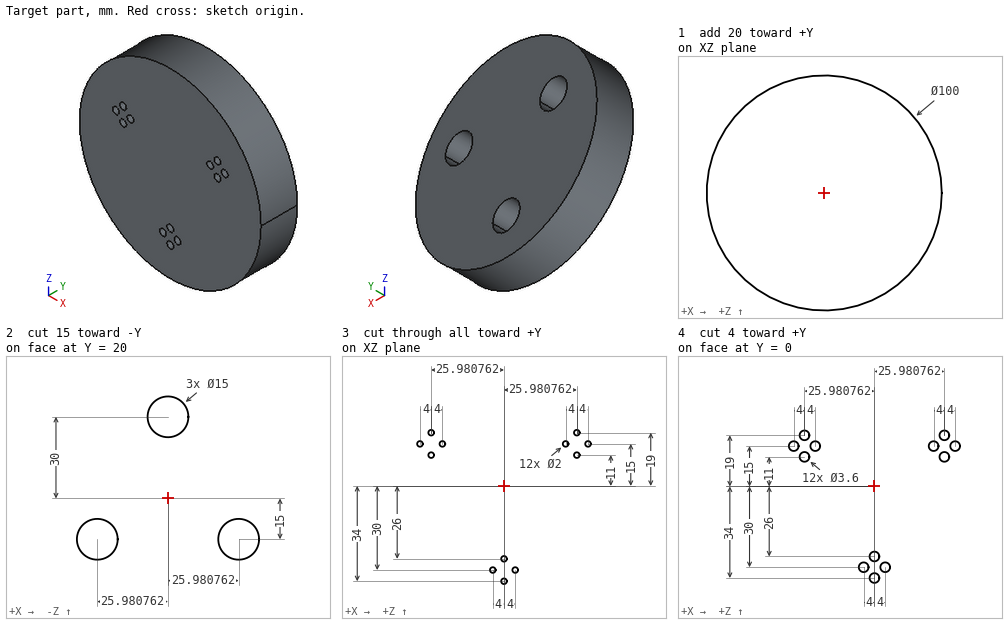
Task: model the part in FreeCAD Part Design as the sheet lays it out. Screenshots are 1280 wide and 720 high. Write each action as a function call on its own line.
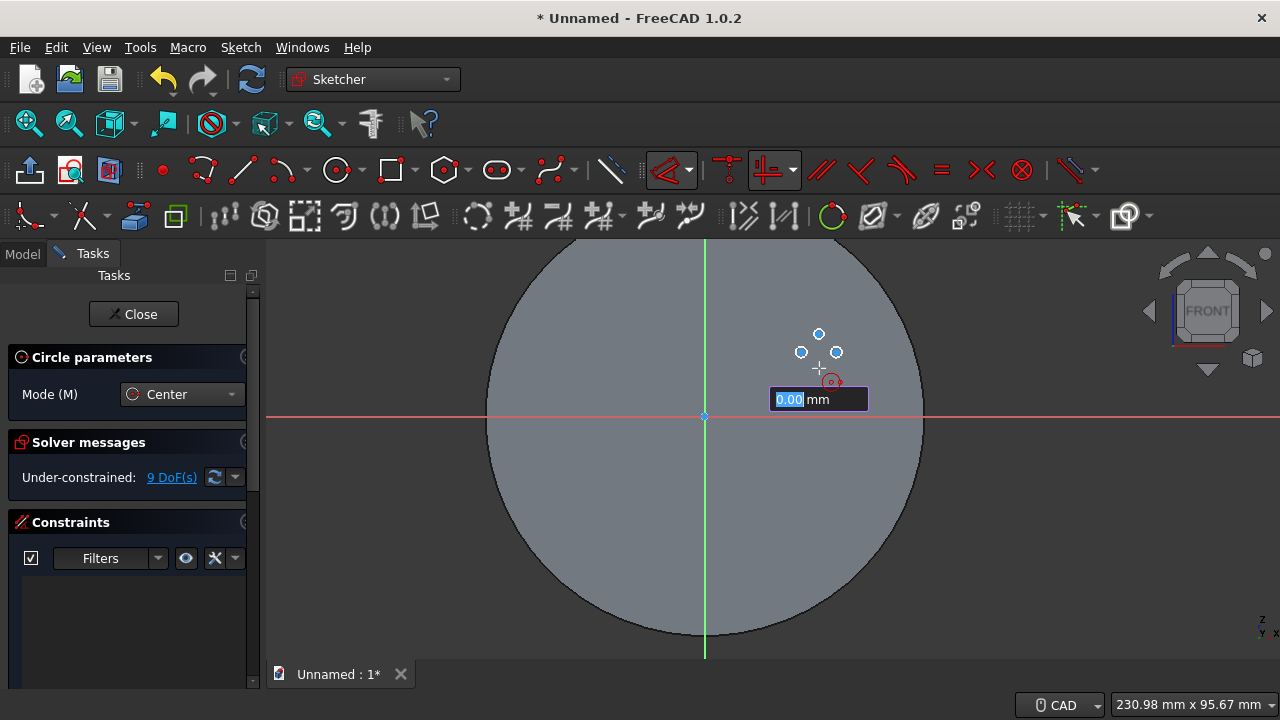
scroll(822, 365, up, 7)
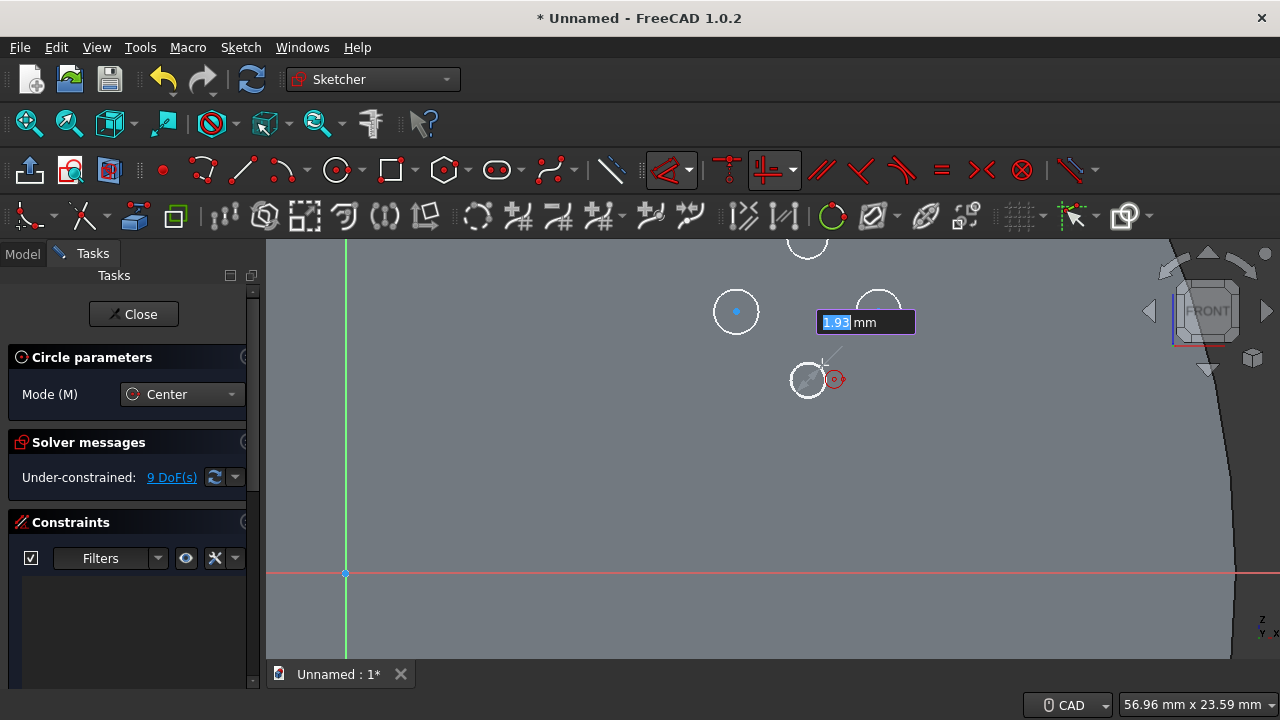
click(821, 365)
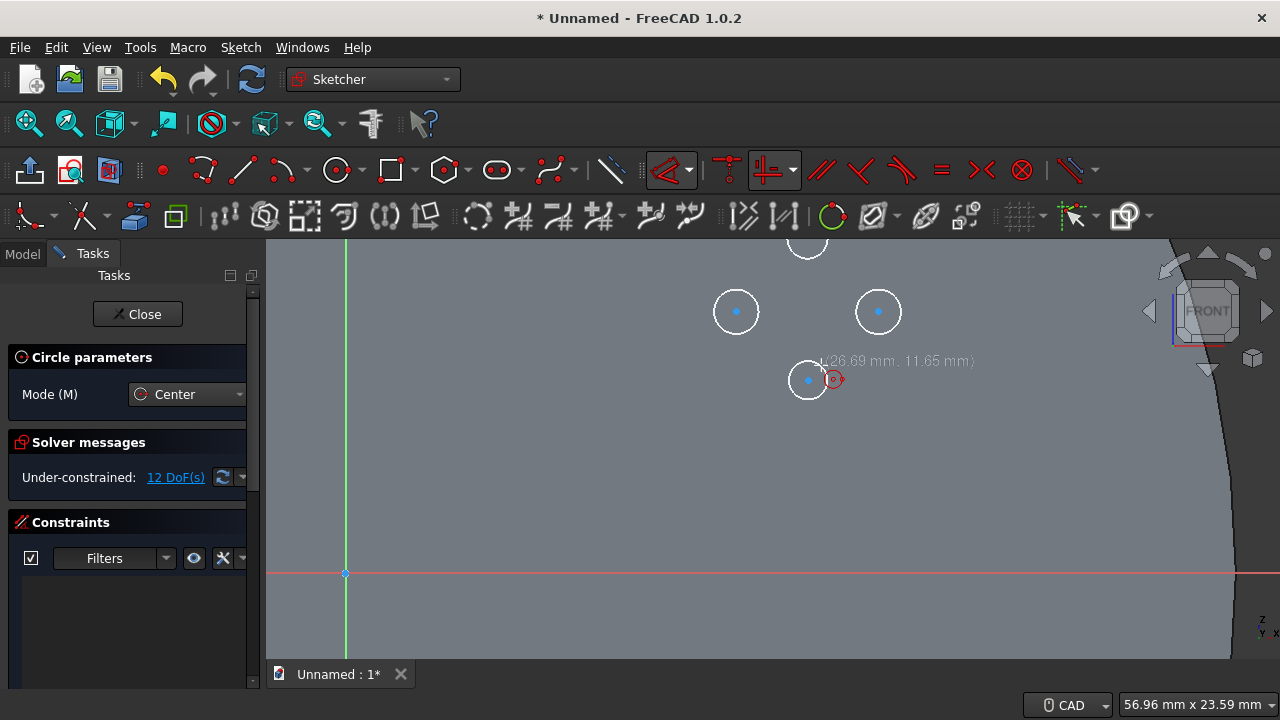
scroll(822, 365, down, 7)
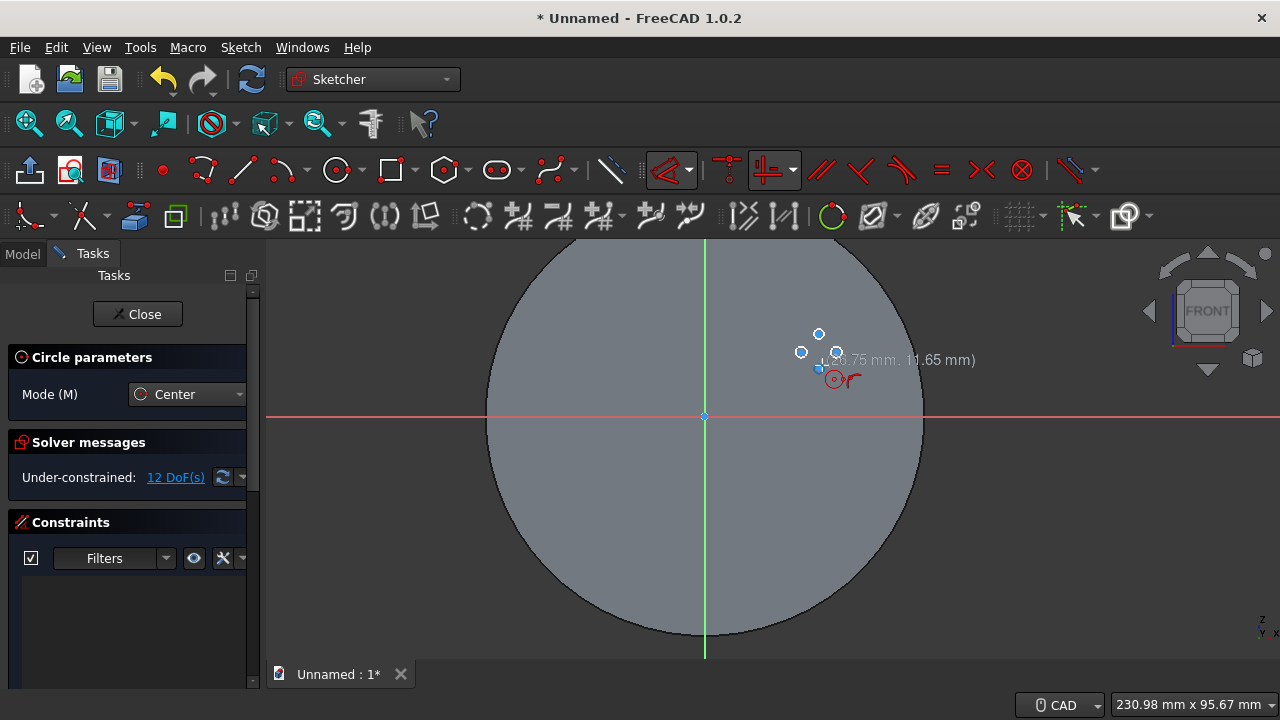
scroll(591, 333, up, 9)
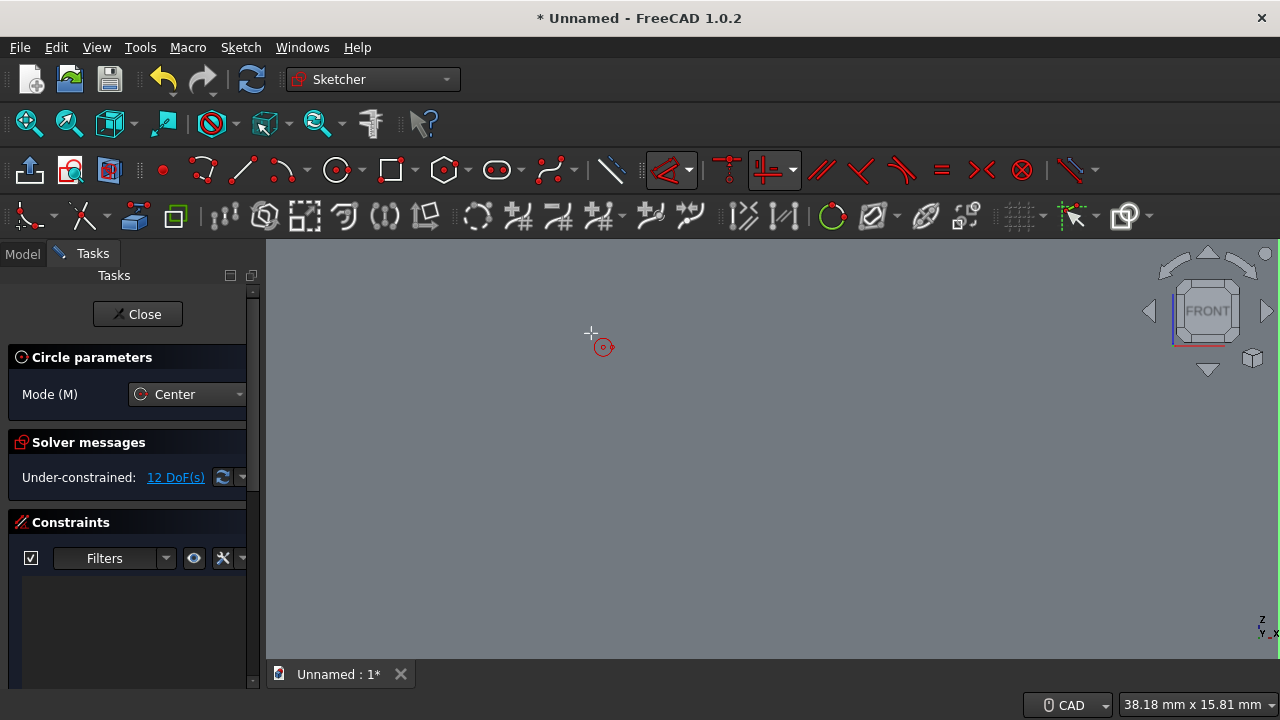
scroll(591, 333, down, 9)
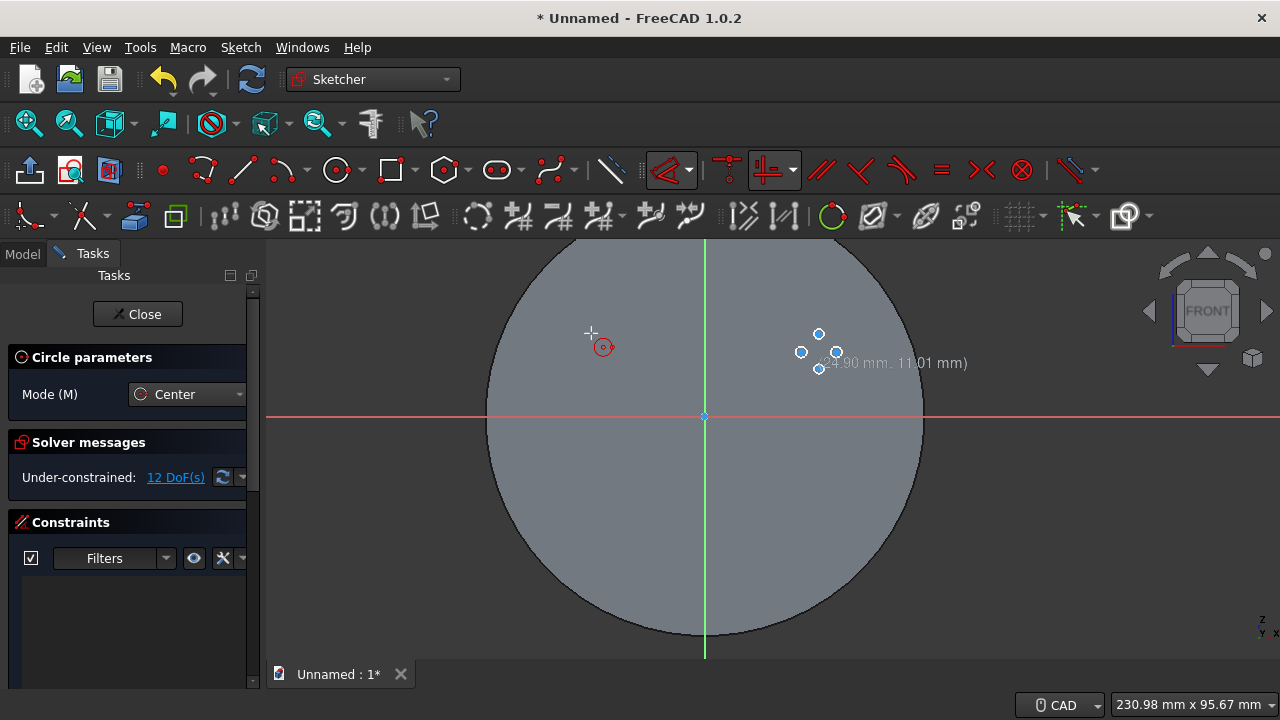
click(591, 333)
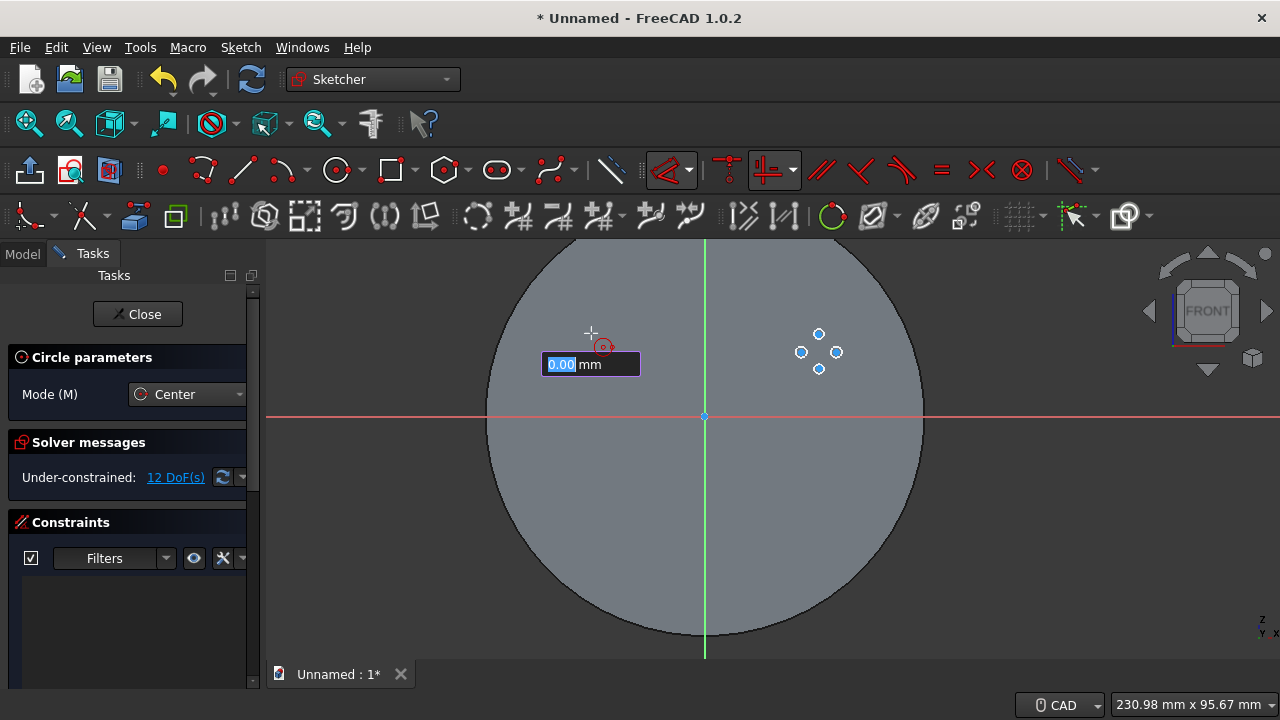
scroll(594, 330, up, 7)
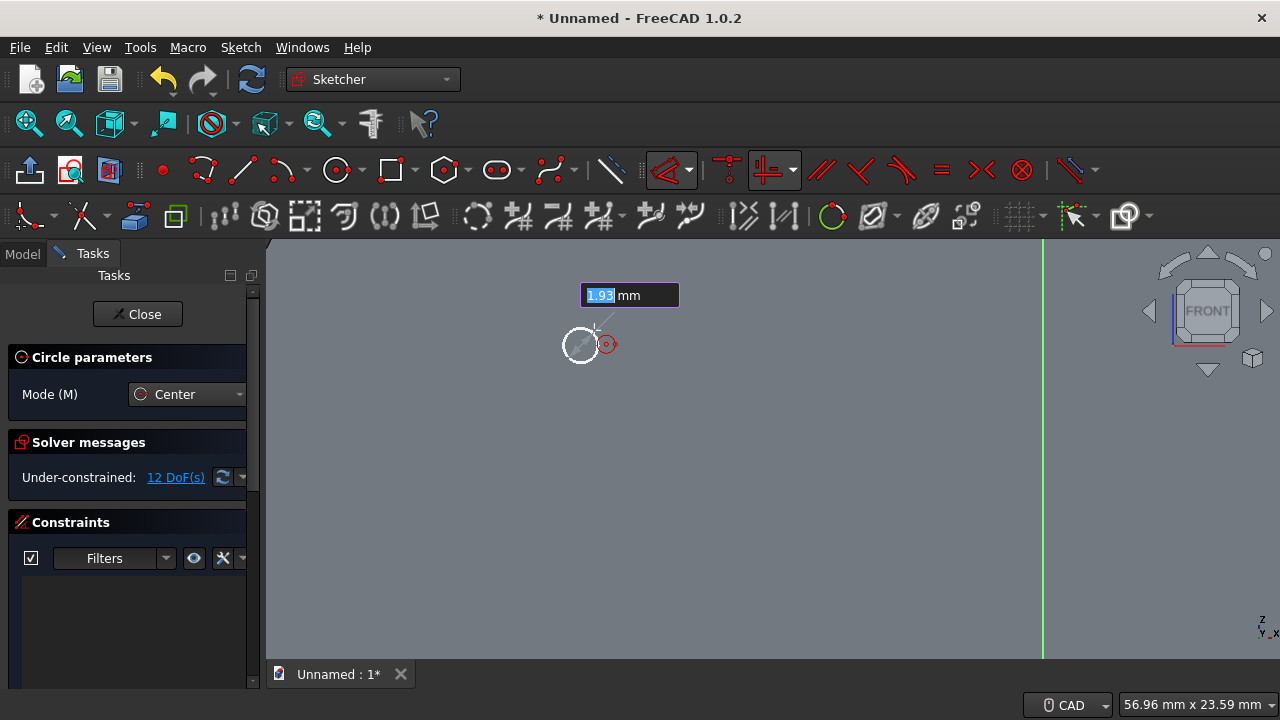
click(593, 330)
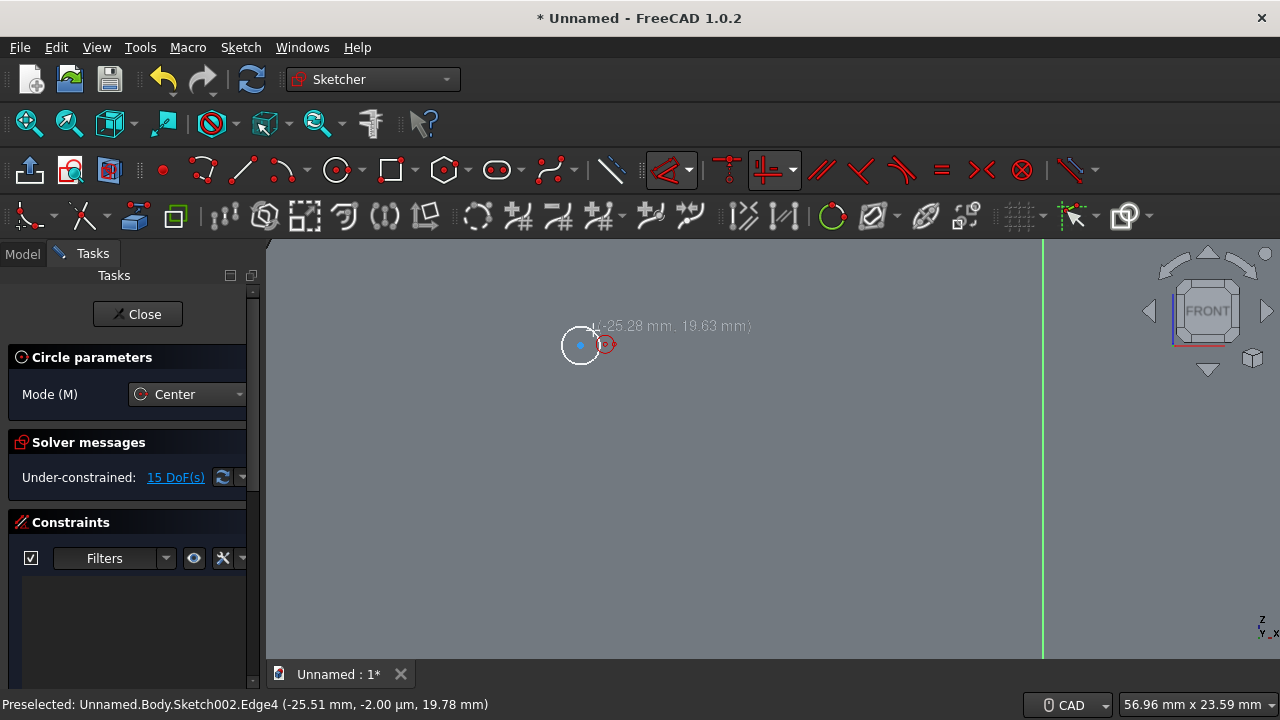
scroll(509, 413, up, 2)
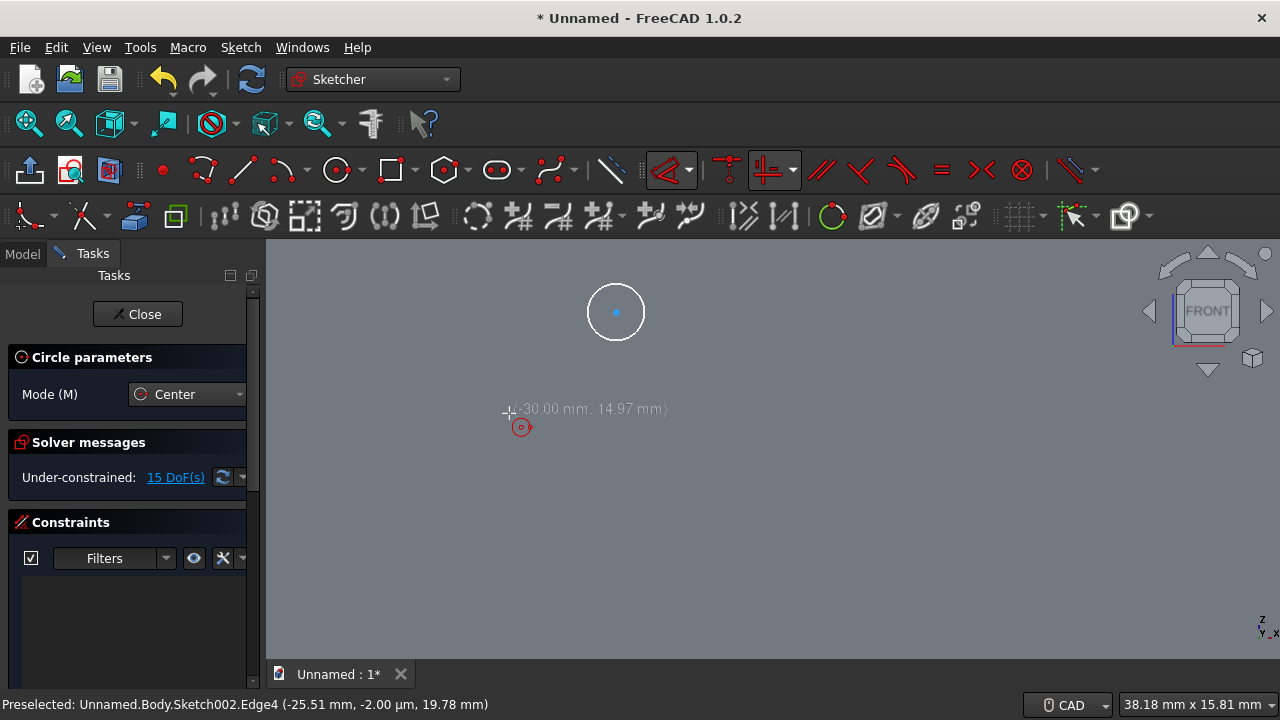
scroll(585, 338, down, 9)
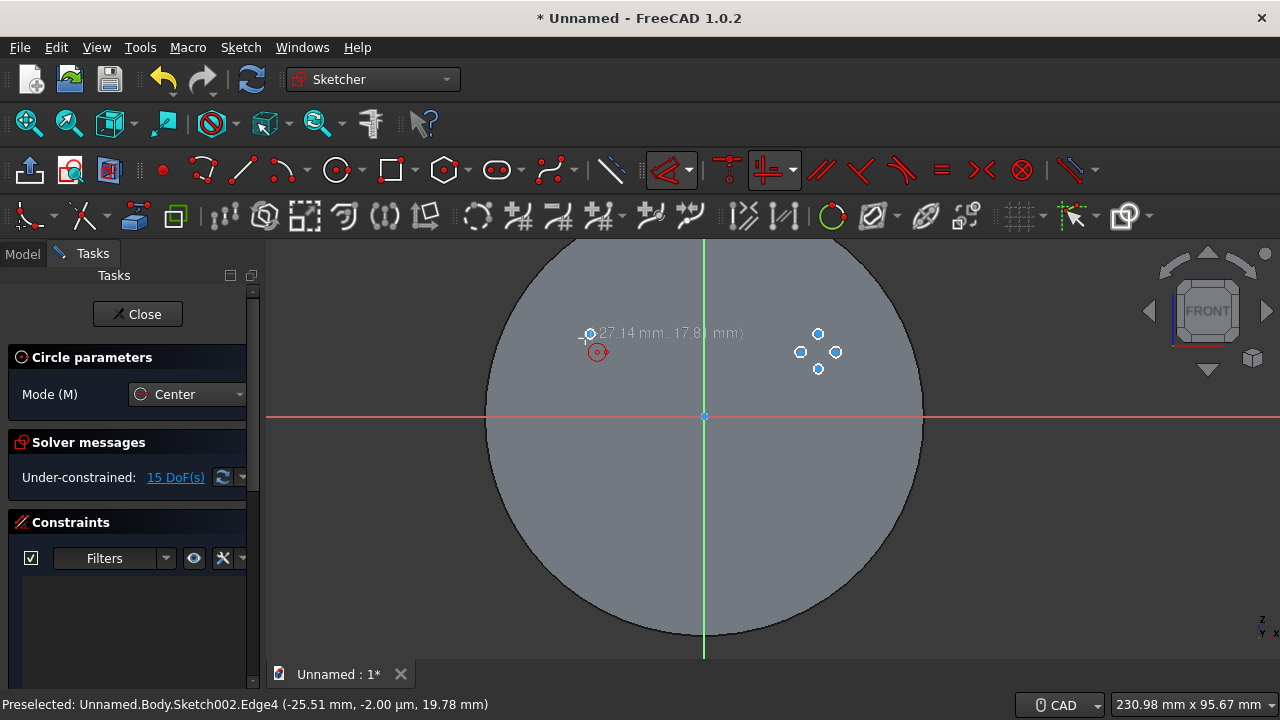
click(573, 351)